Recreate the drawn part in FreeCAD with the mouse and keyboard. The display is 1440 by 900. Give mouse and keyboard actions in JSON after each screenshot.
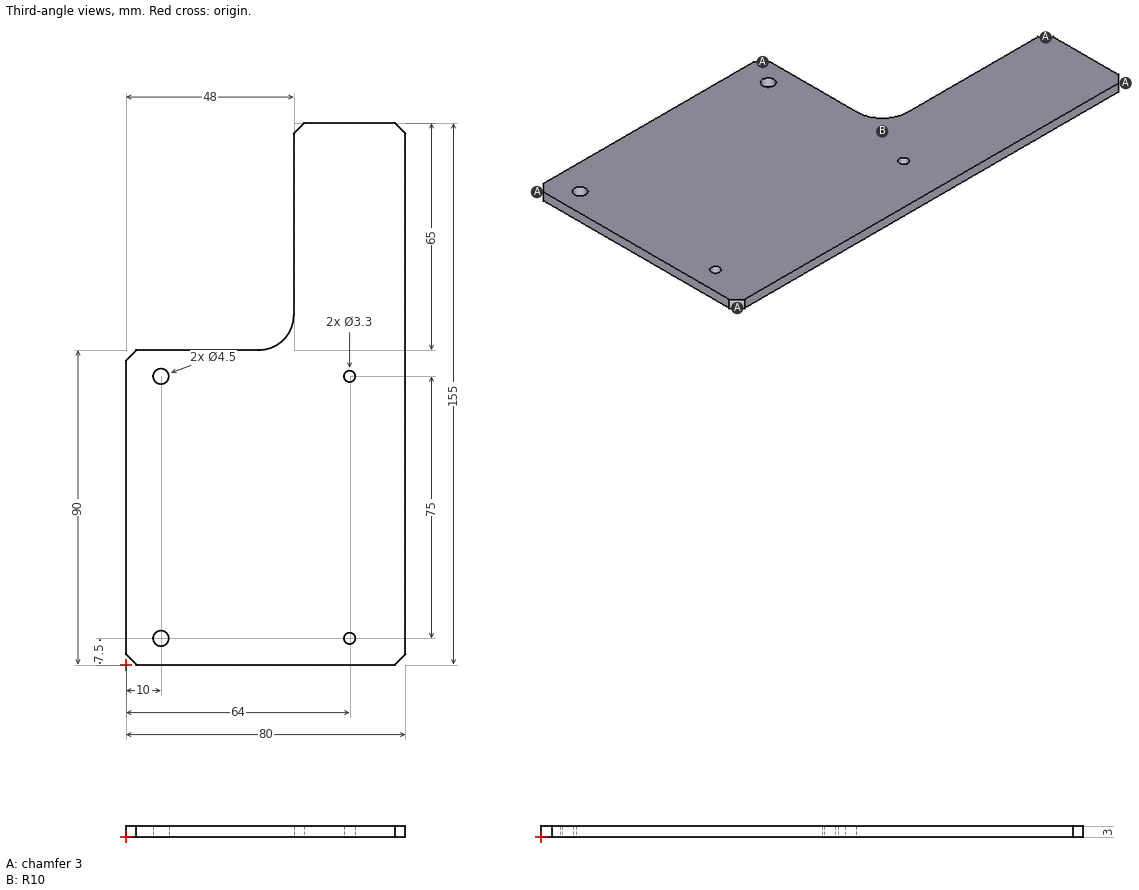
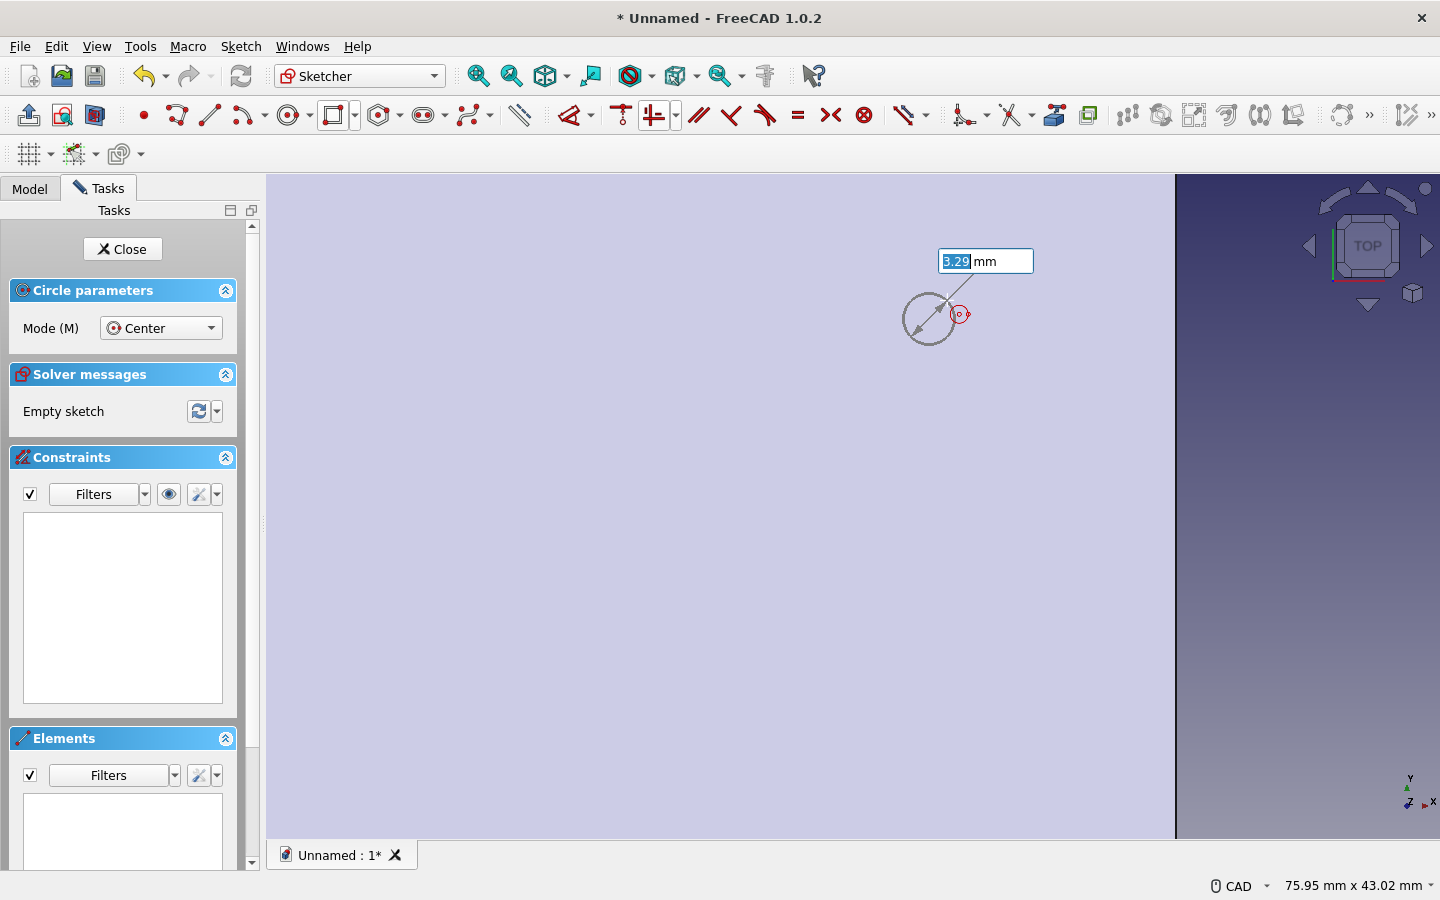
{"action": "type", "text": "3.3"}
{"action": "key", "text": "Return"}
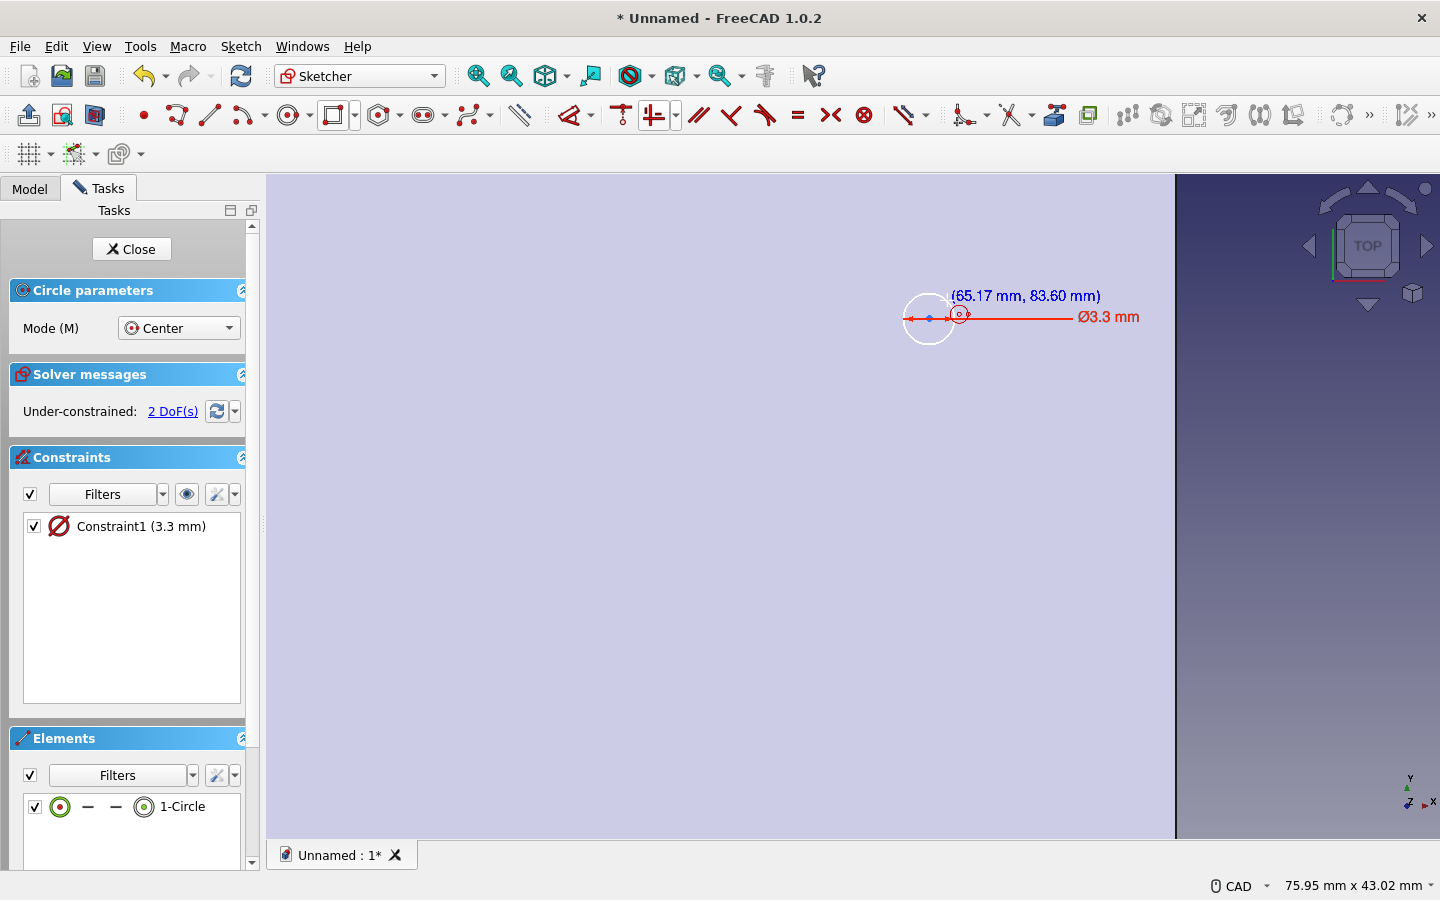
{"action": "scroll", "coordinate": [930, 318], "scroll_direction": "down", "scroll_amount": 6}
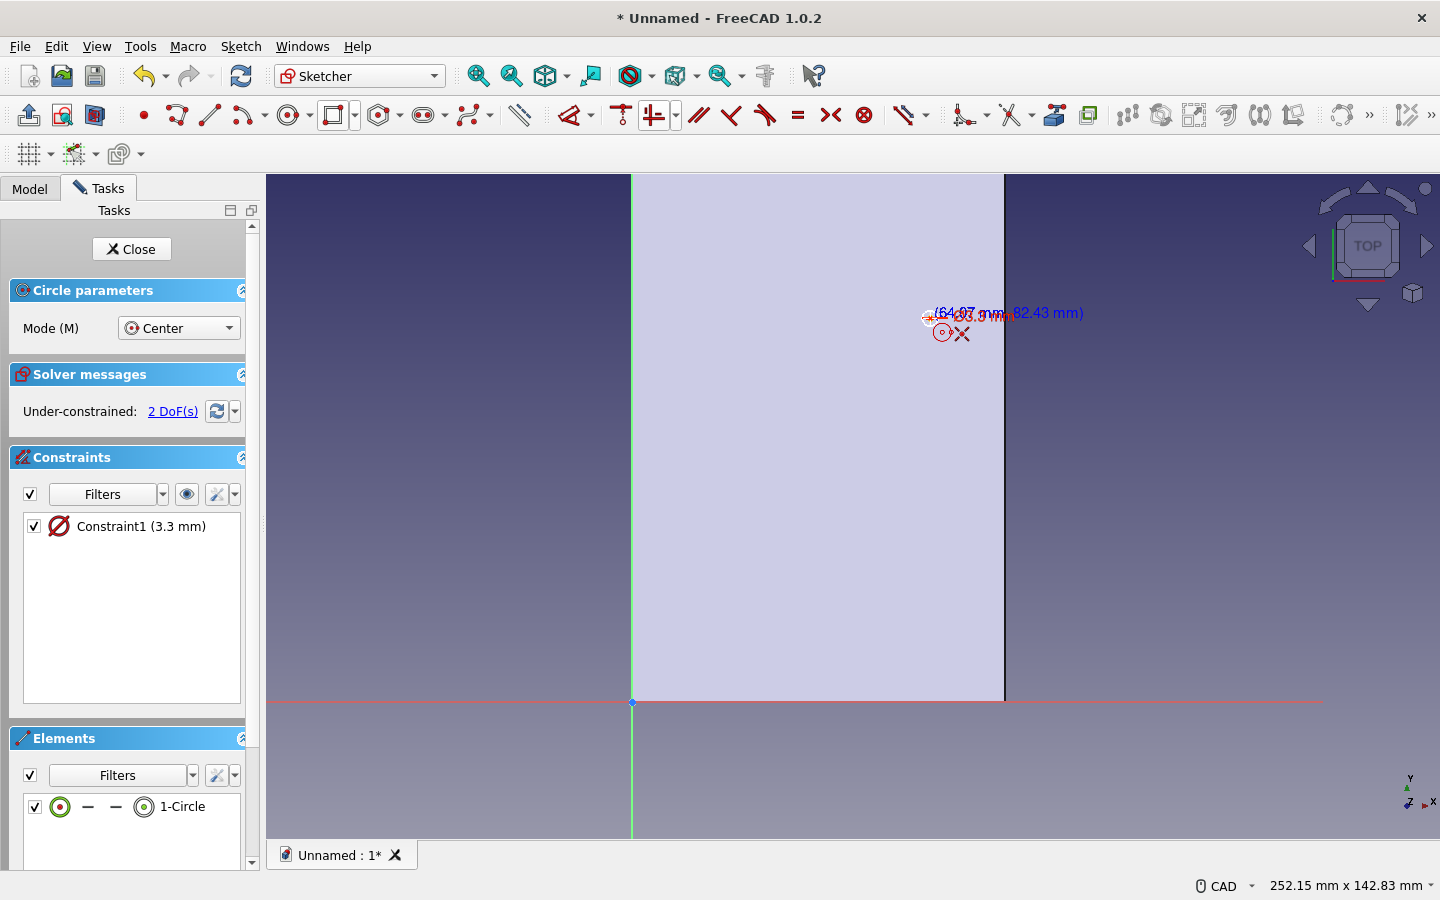
{"action": "scroll", "coordinate": [930, 667], "scroll_direction": "up", "scroll_amount": 6}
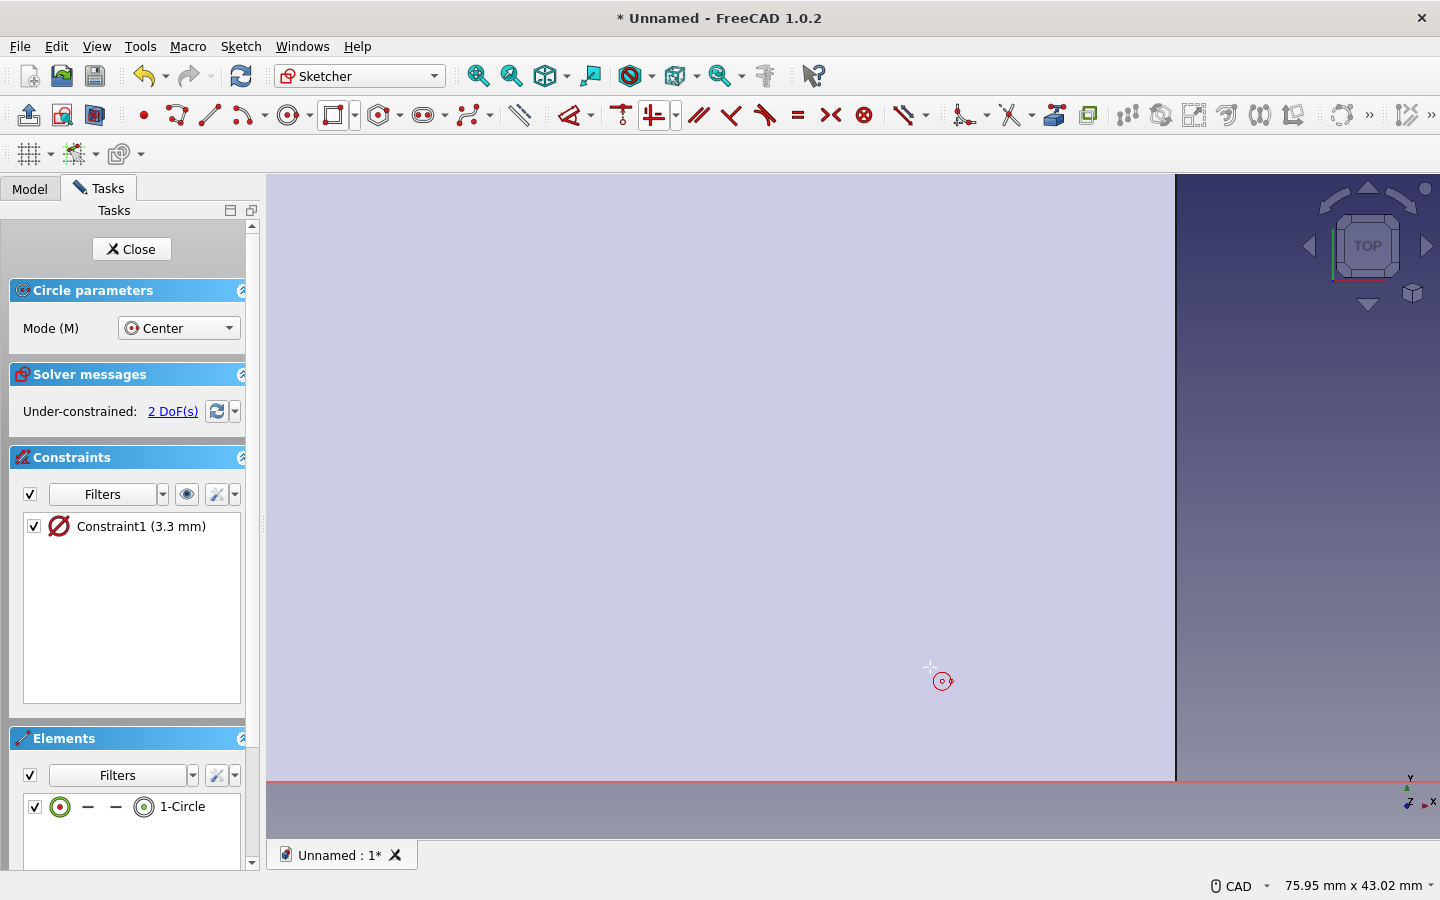
{"action": "left_click", "coordinate": [929, 666]}
{"action": "mouse_move", "coordinate": [947, 648]}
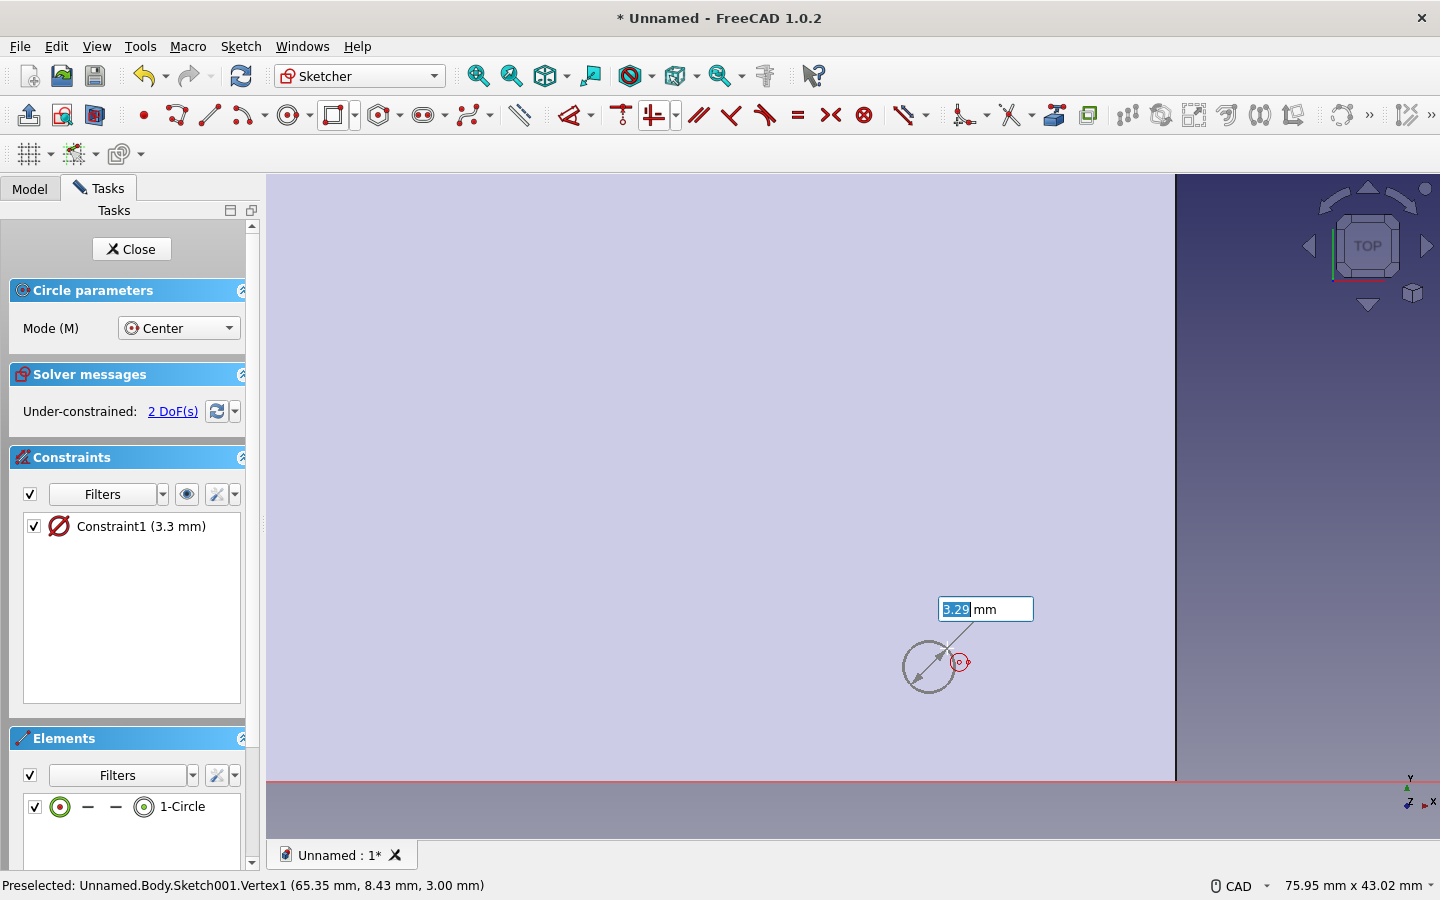
{"action": "type", "text": "3.3"}
{"action": "key", "text": "Return"}
{"action": "key", "text": "Escape"}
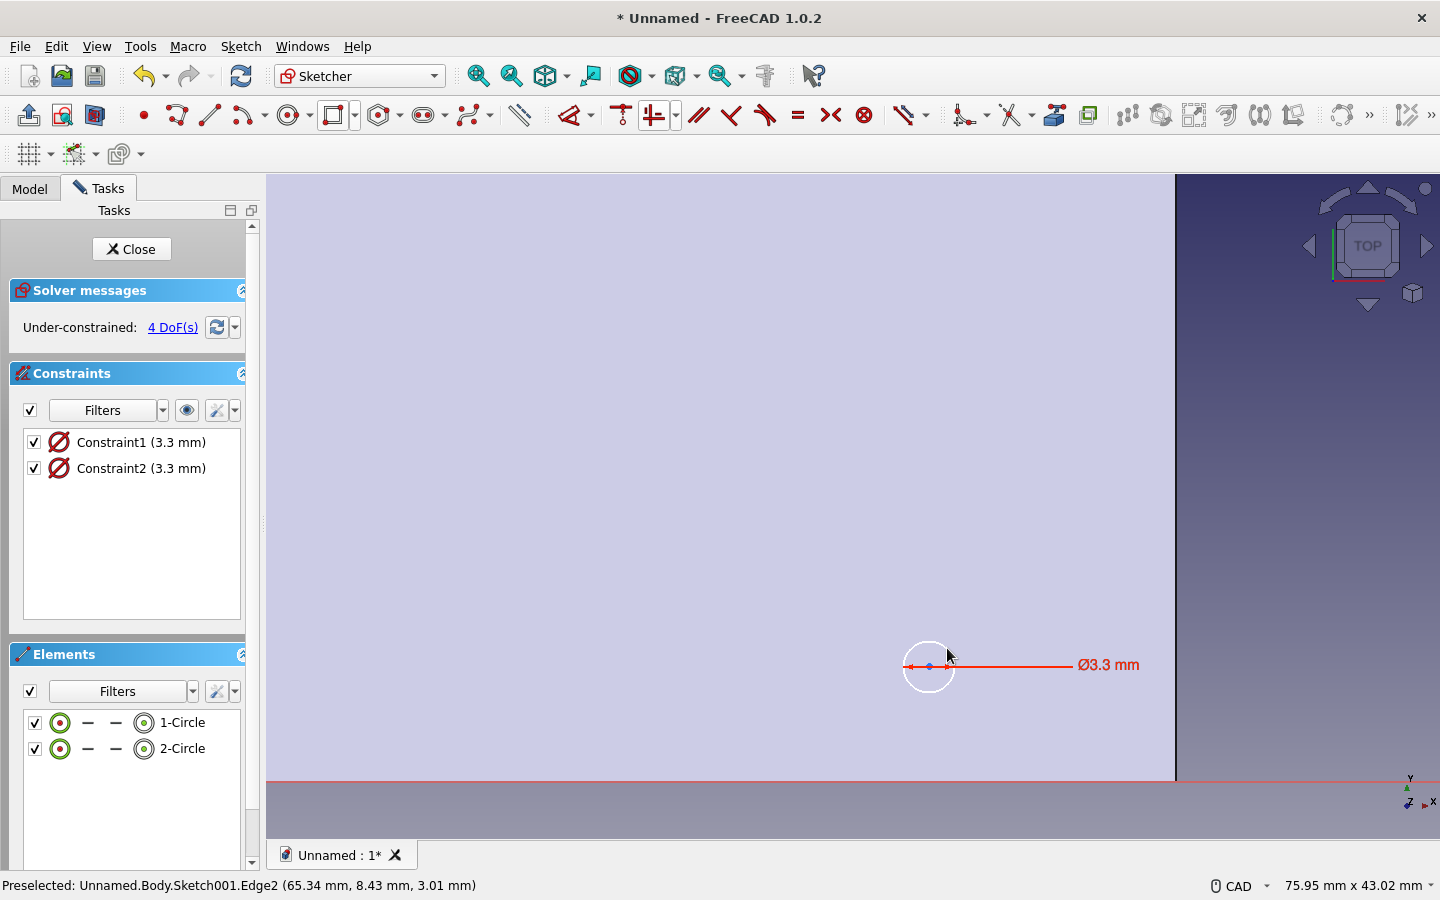
{"action": "scroll", "coordinate": [930, 668], "scroll_direction": "down", "scroll_amount": 6}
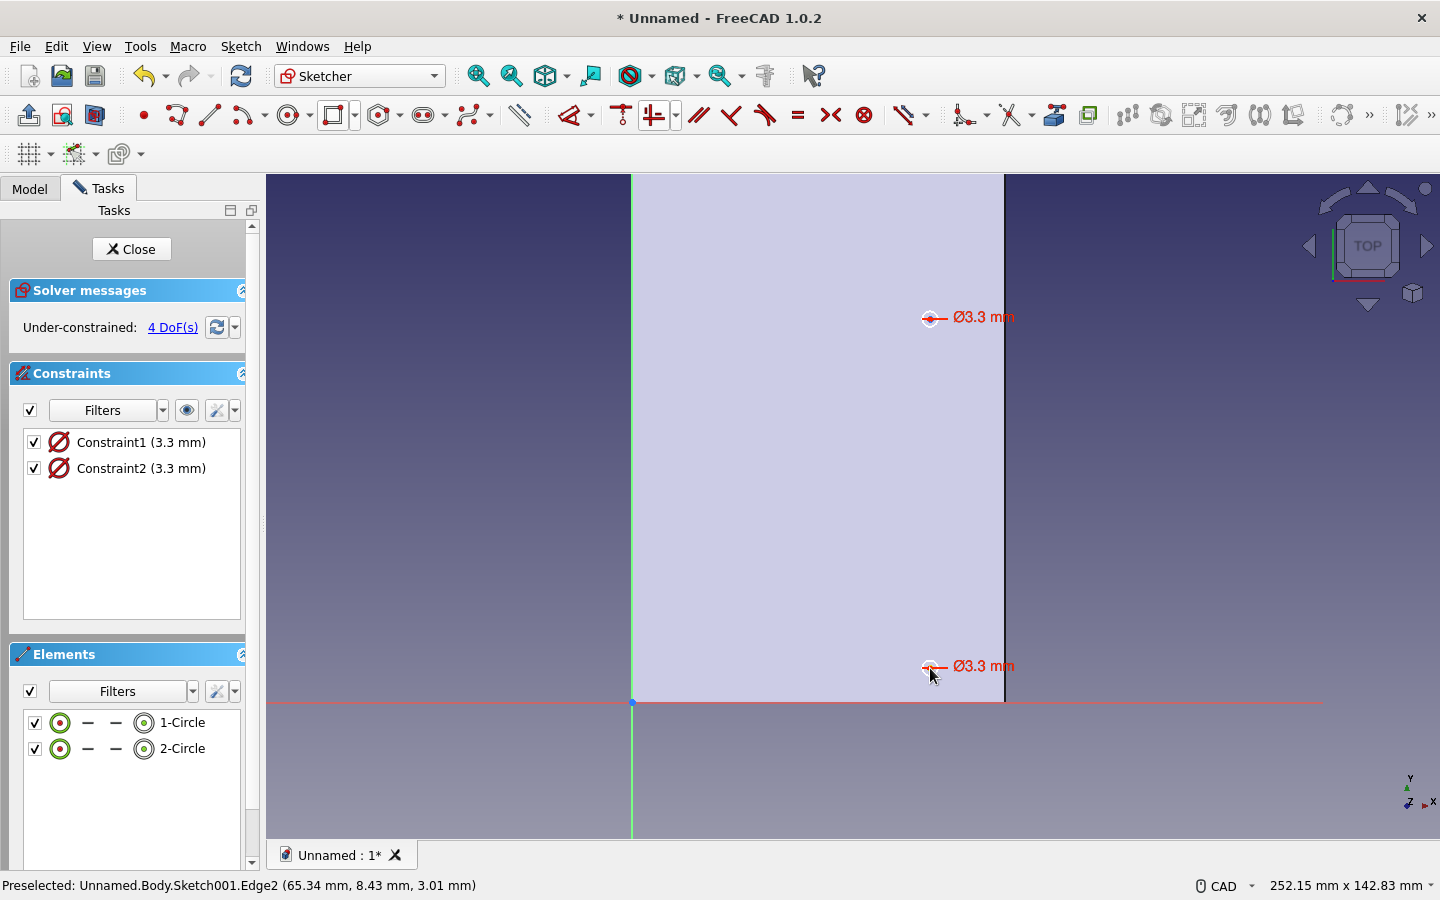
{"action": "left_click", "coordinate": [930, 319]}